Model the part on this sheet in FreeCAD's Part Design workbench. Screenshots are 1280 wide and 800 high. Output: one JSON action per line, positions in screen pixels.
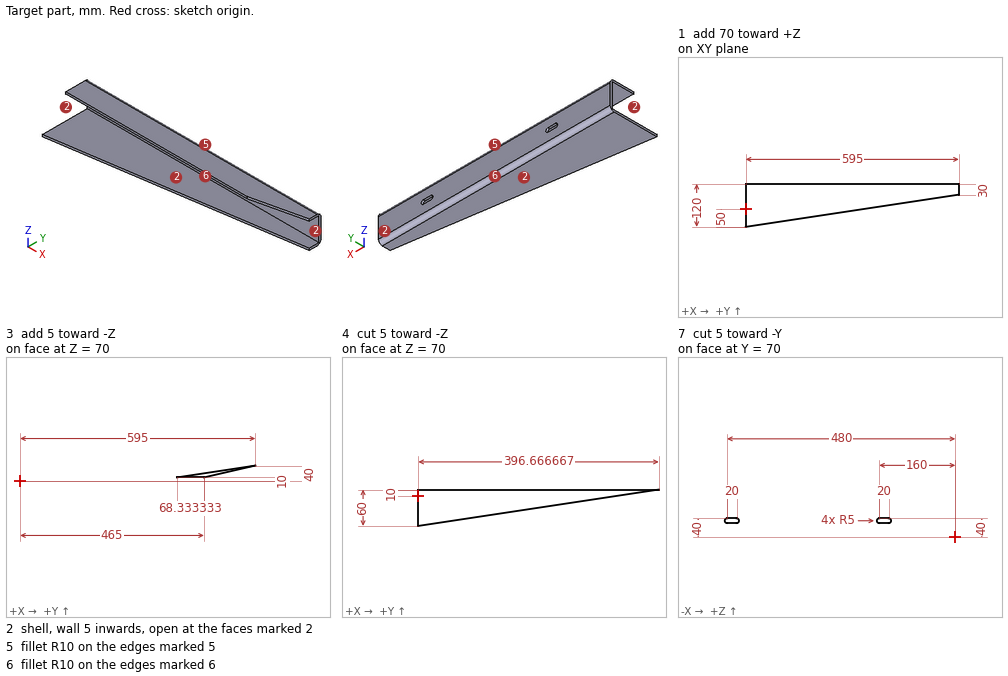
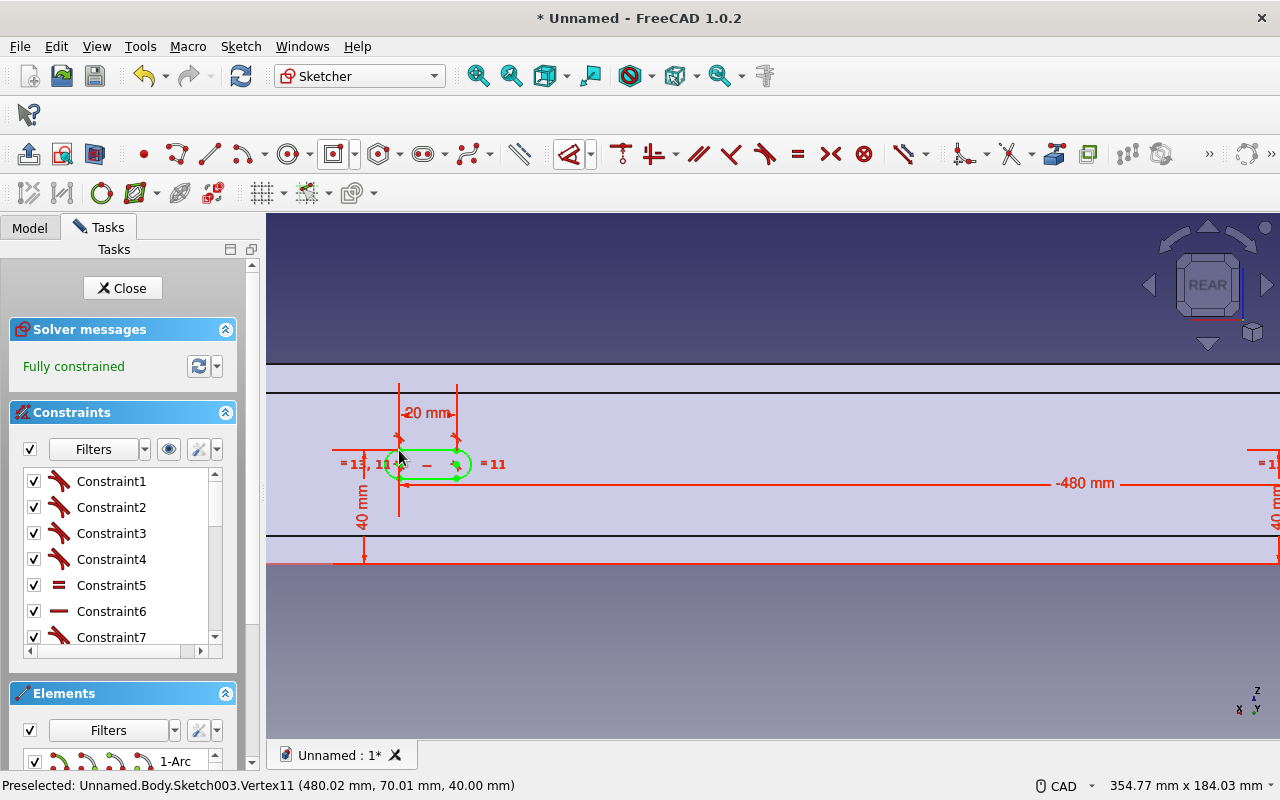
{"action": "left_click", "coordinate": [123, 288]}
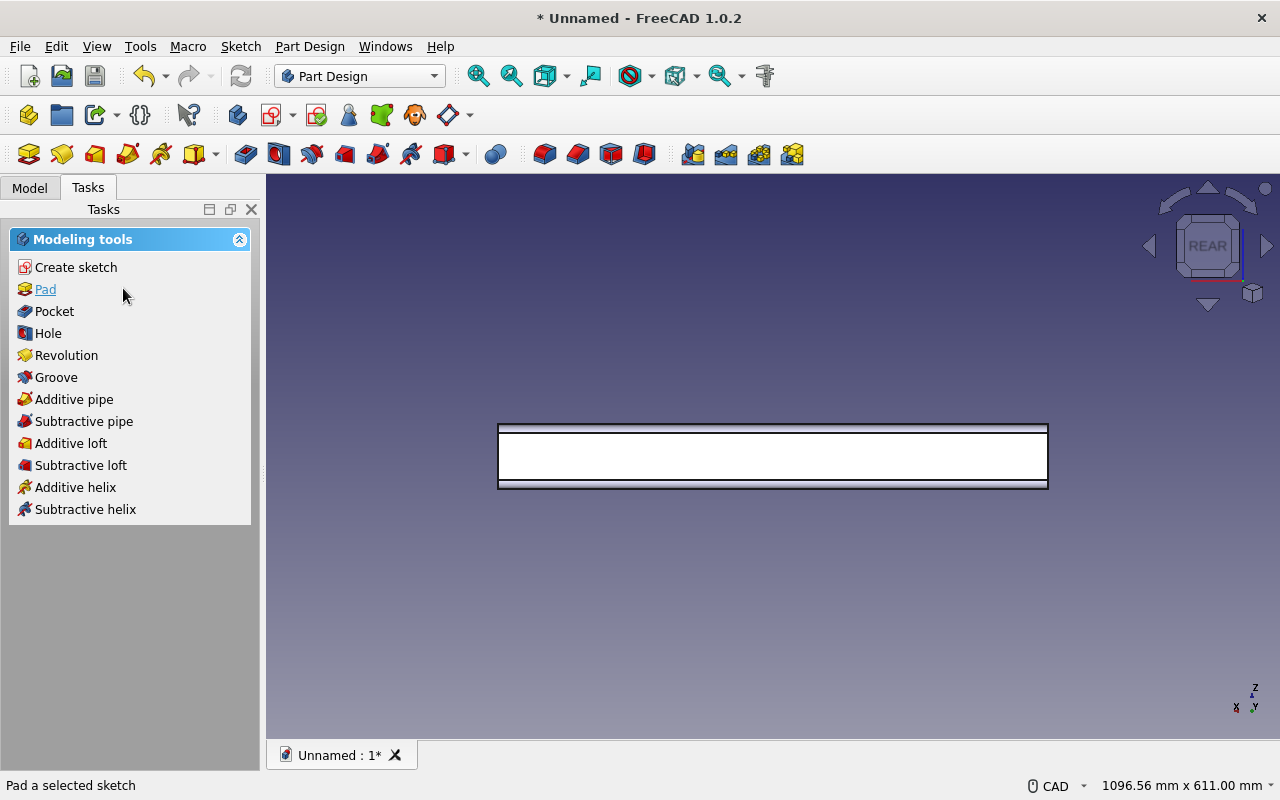
{"action": "left_click", "coordinate": [246, 154]}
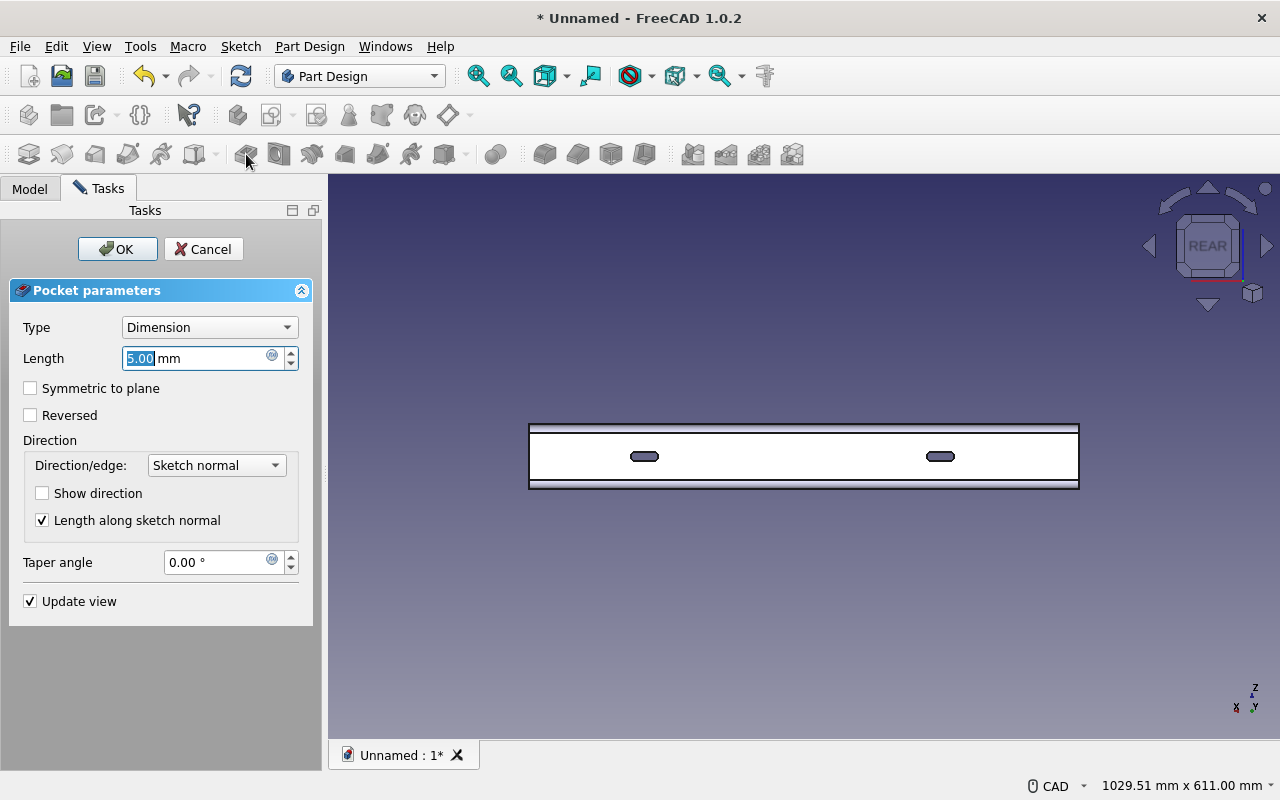
{"action": "type", "text": "5"}
{"action": "key", "text": "Tab"}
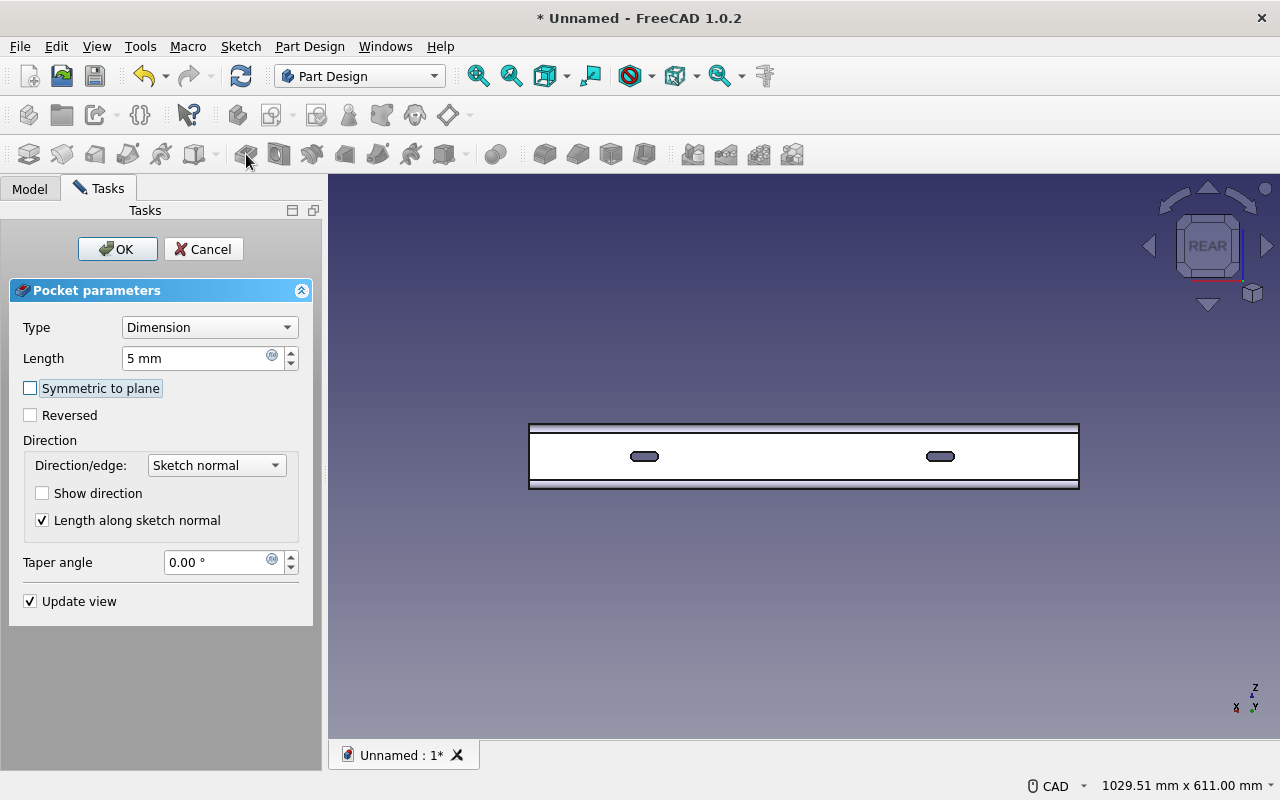
{"action": "left_click", "coordinate": [118, 249]}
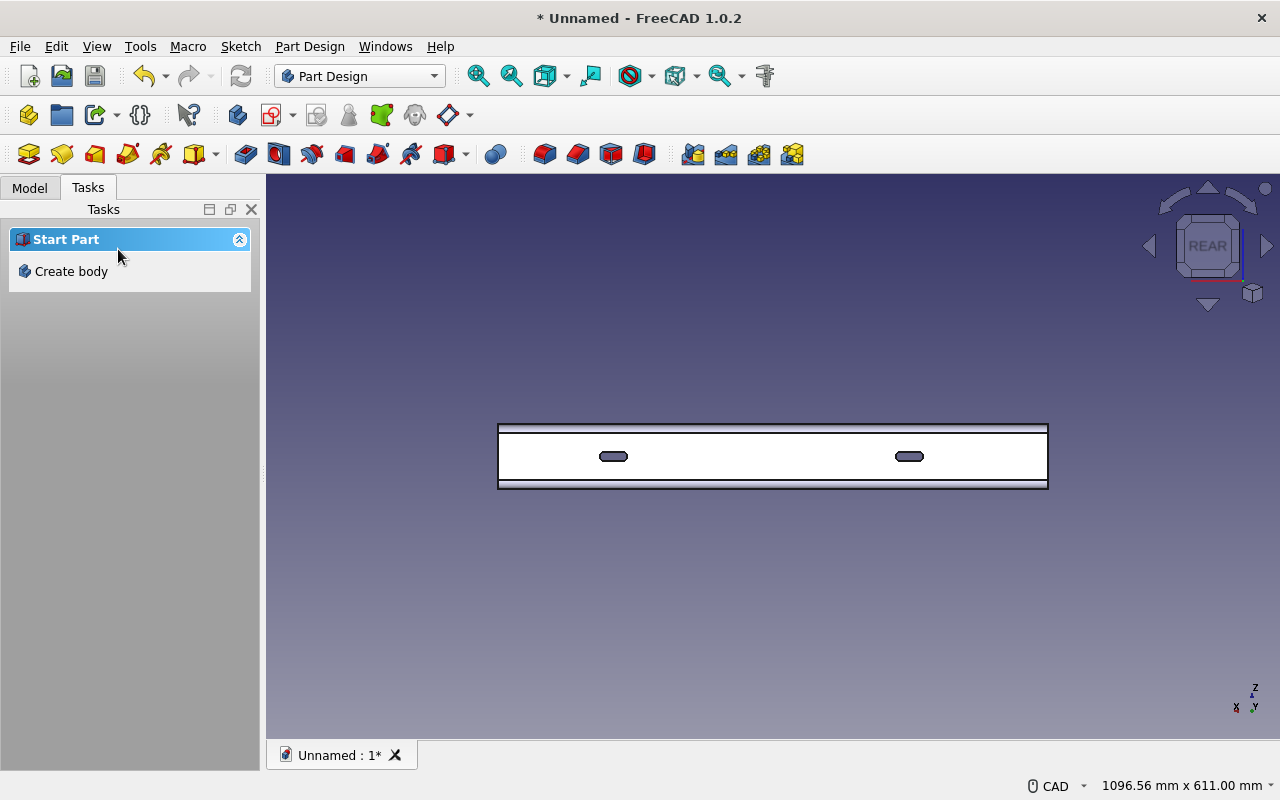
{"action": "key", "text": "0"}